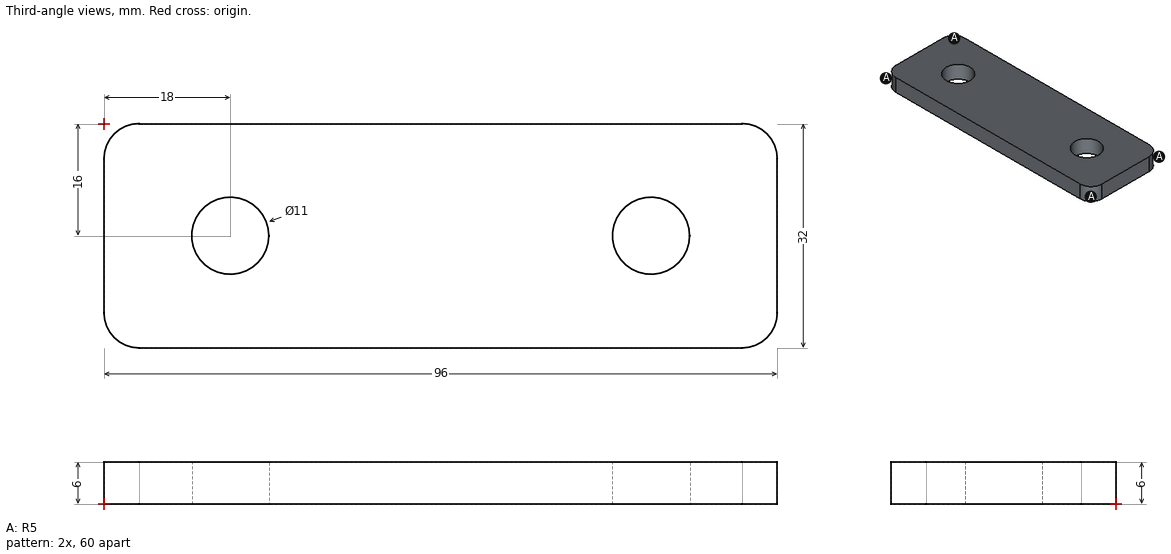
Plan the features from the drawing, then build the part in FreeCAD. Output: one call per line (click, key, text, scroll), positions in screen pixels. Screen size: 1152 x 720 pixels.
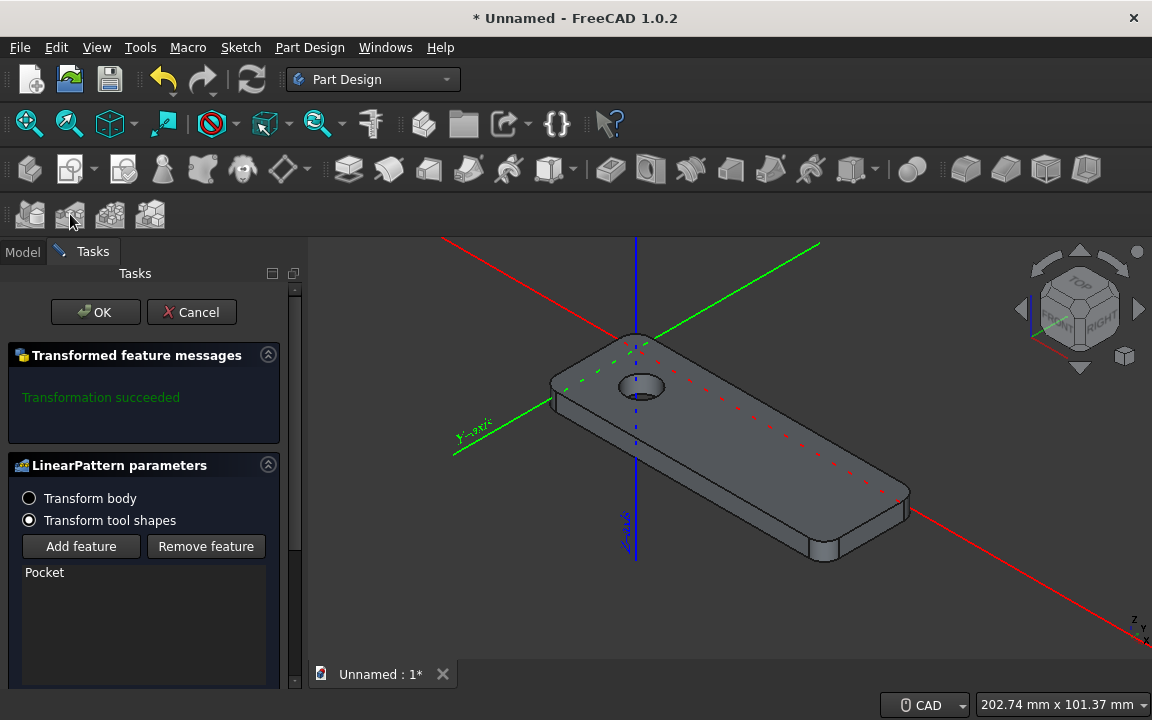
scroll(295, 486, down, 2)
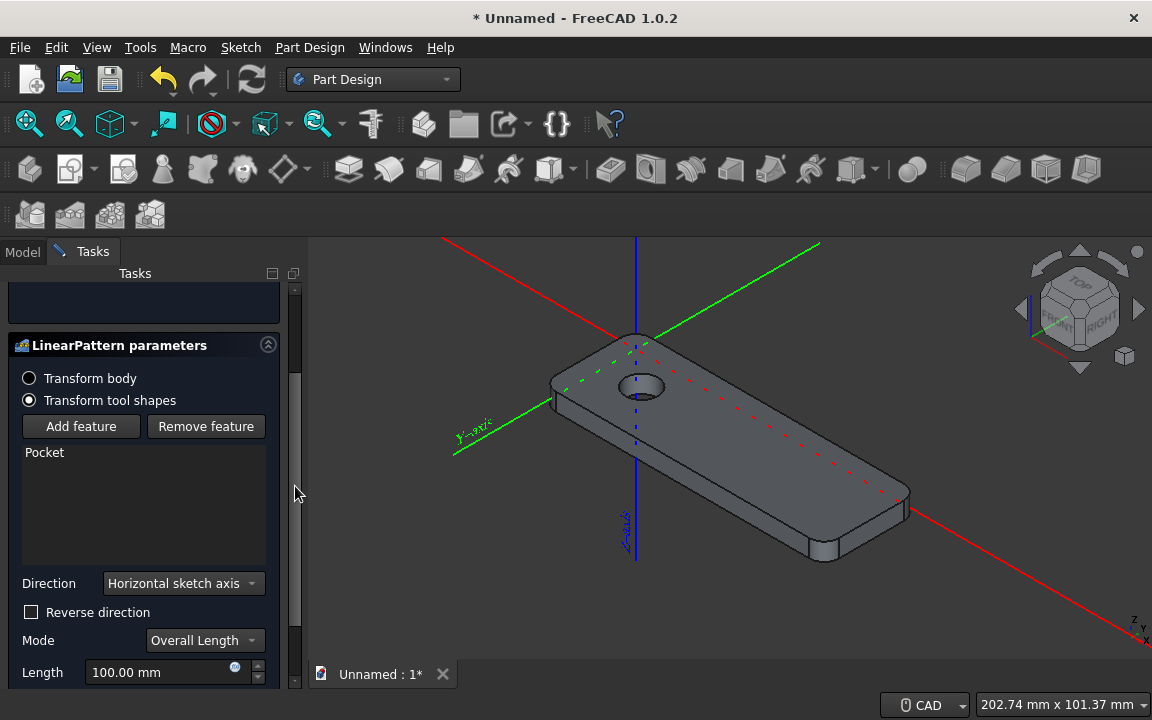
click(184, 584)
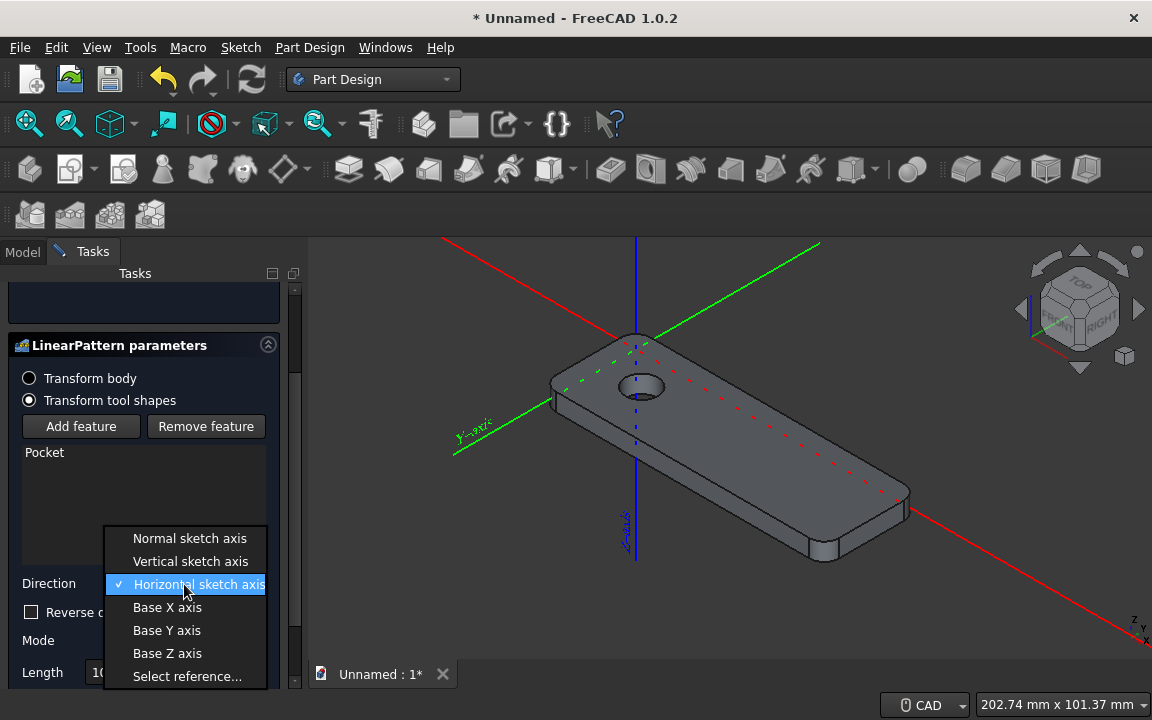
click(184, 608)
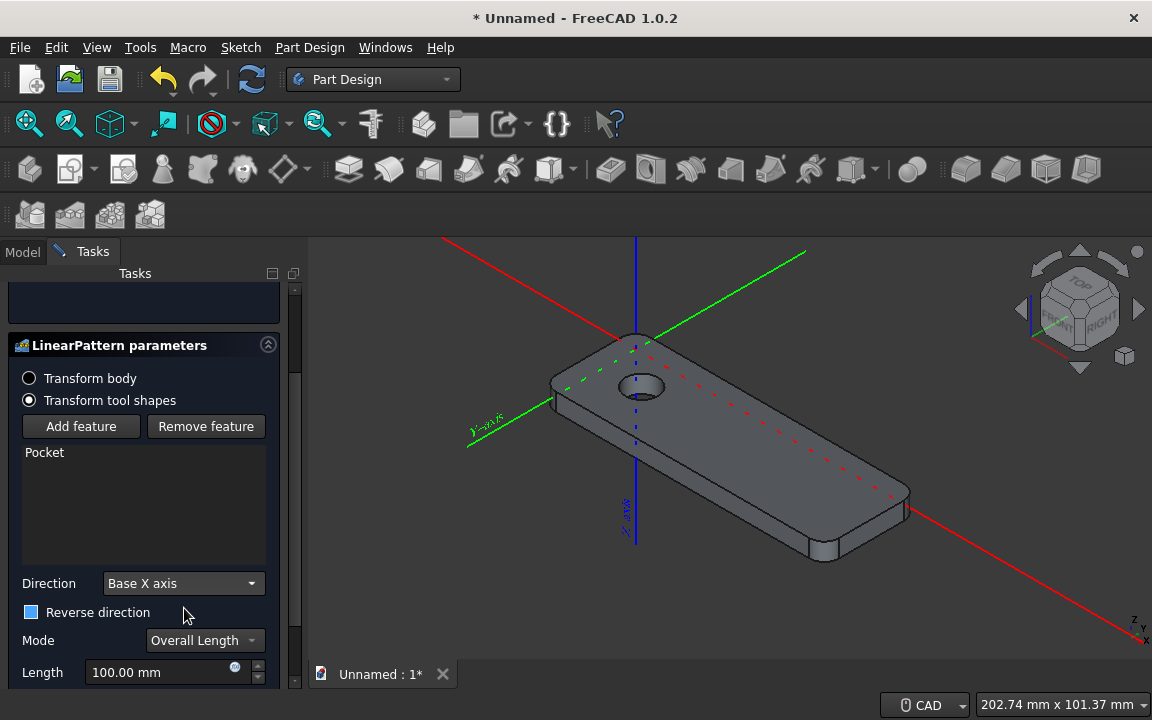
click(206, 640)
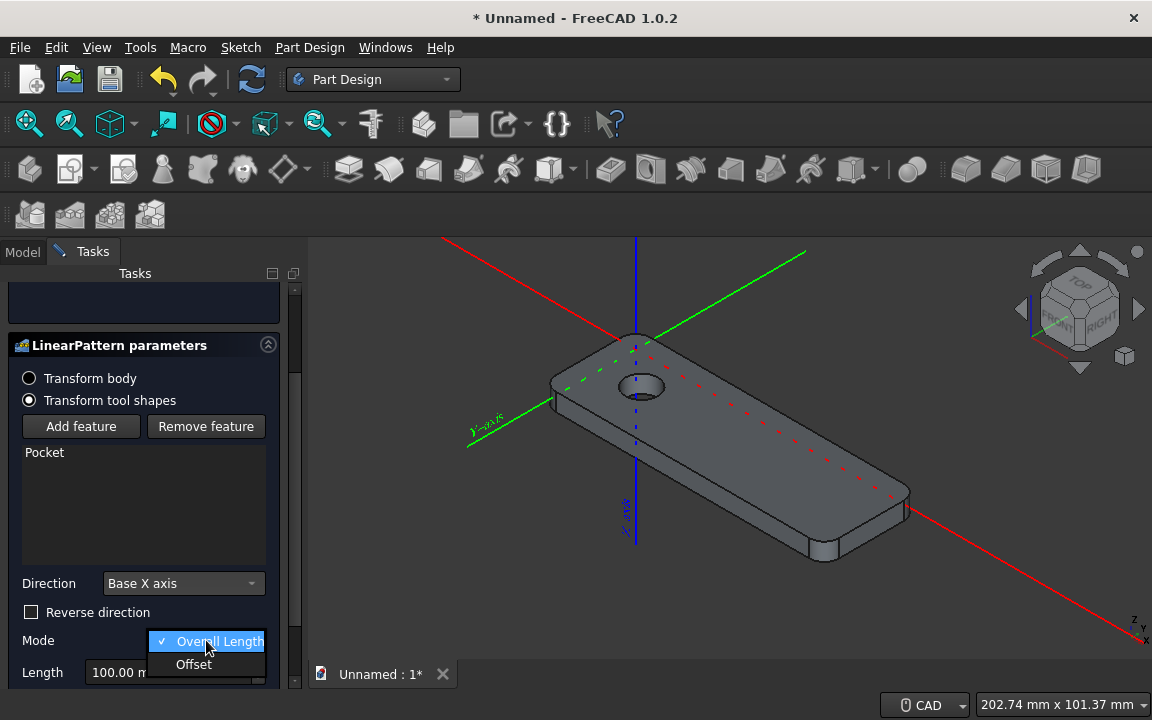
click(206, 664)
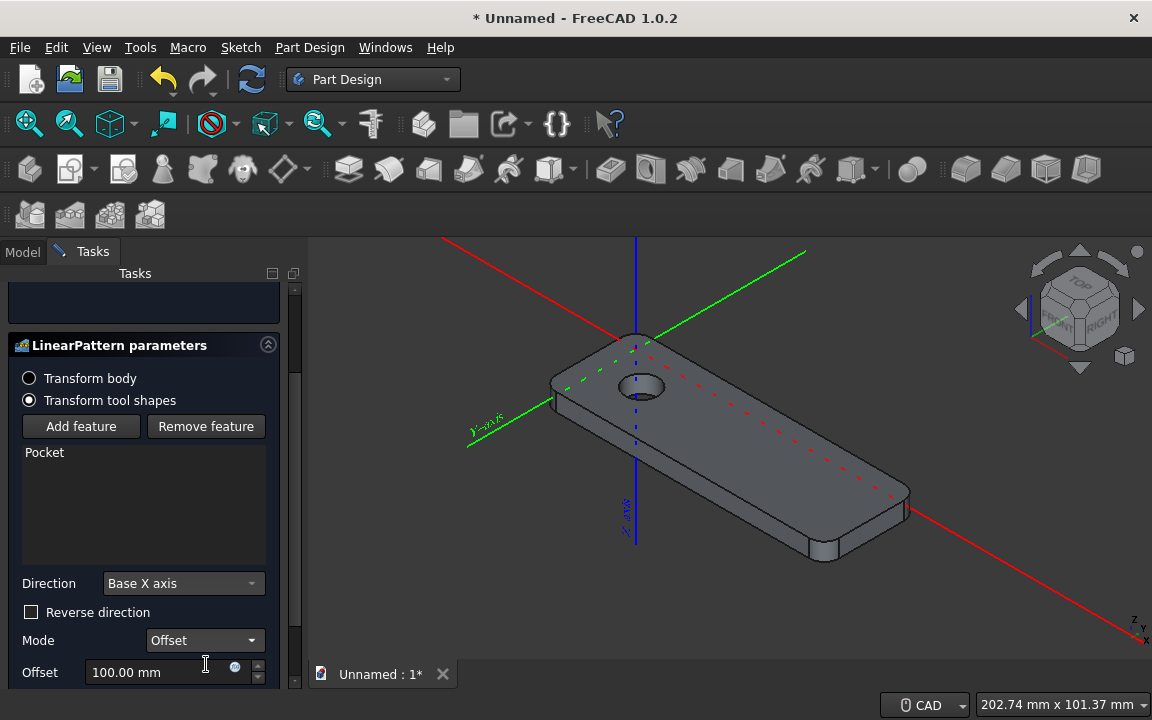
triple_click(168, 672)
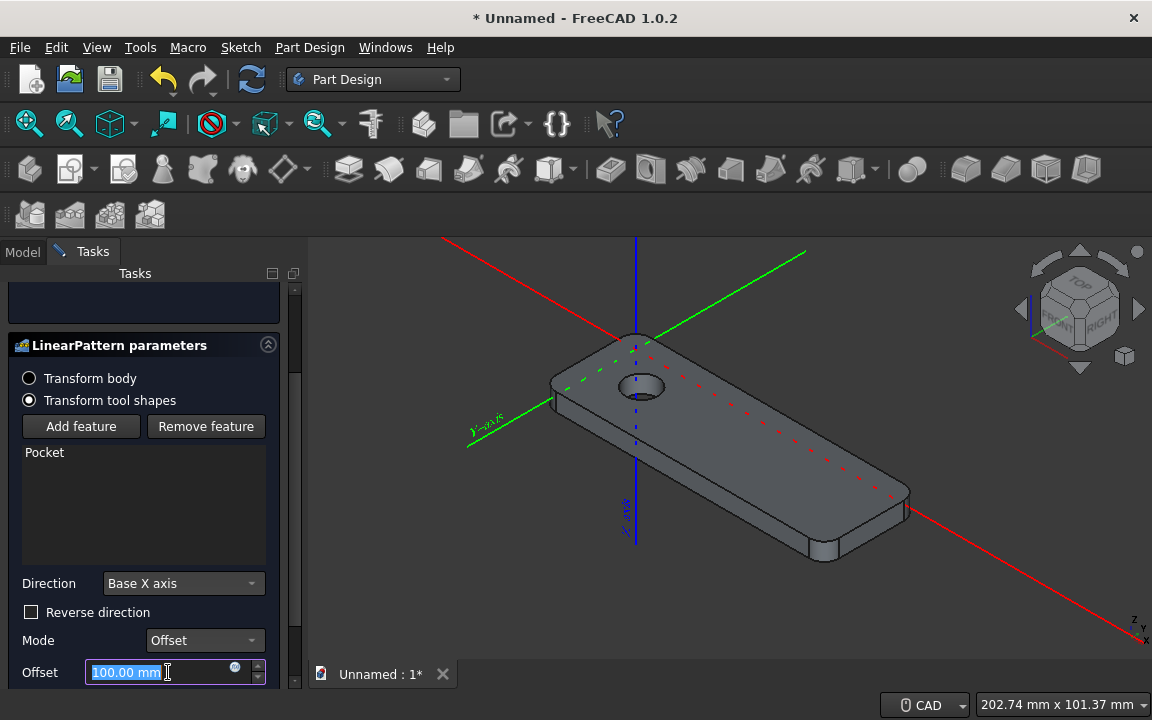
text(60)
key(Tab)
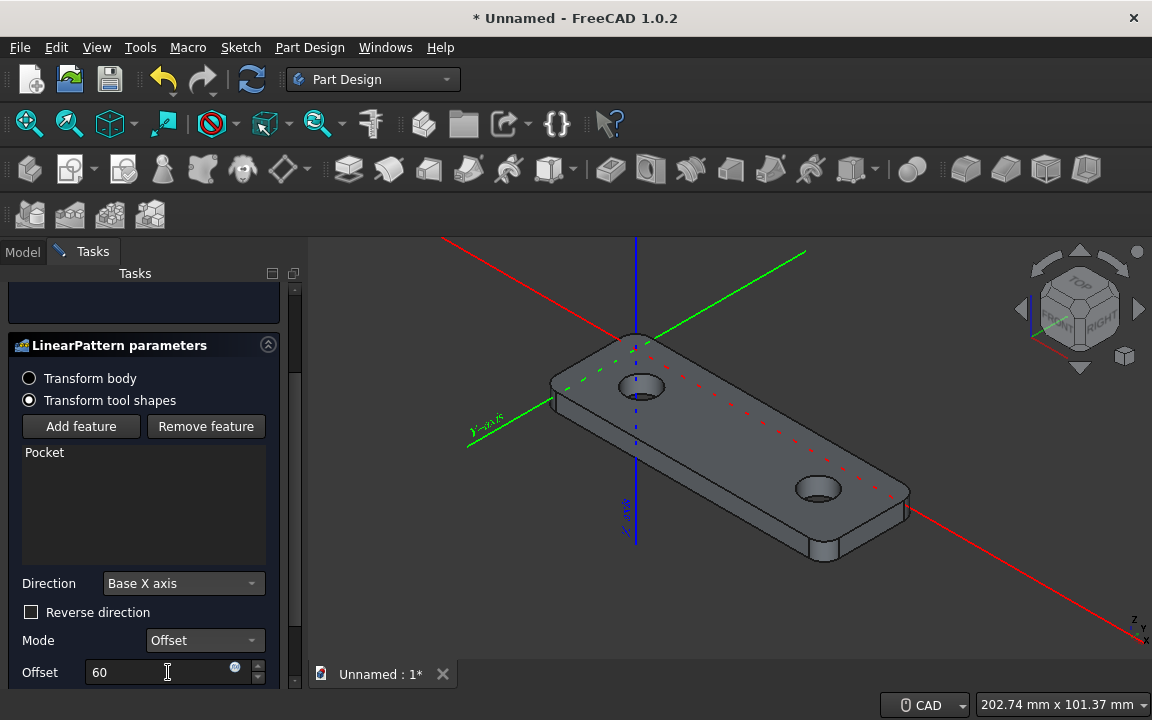
scroll(295, 486, down, 2)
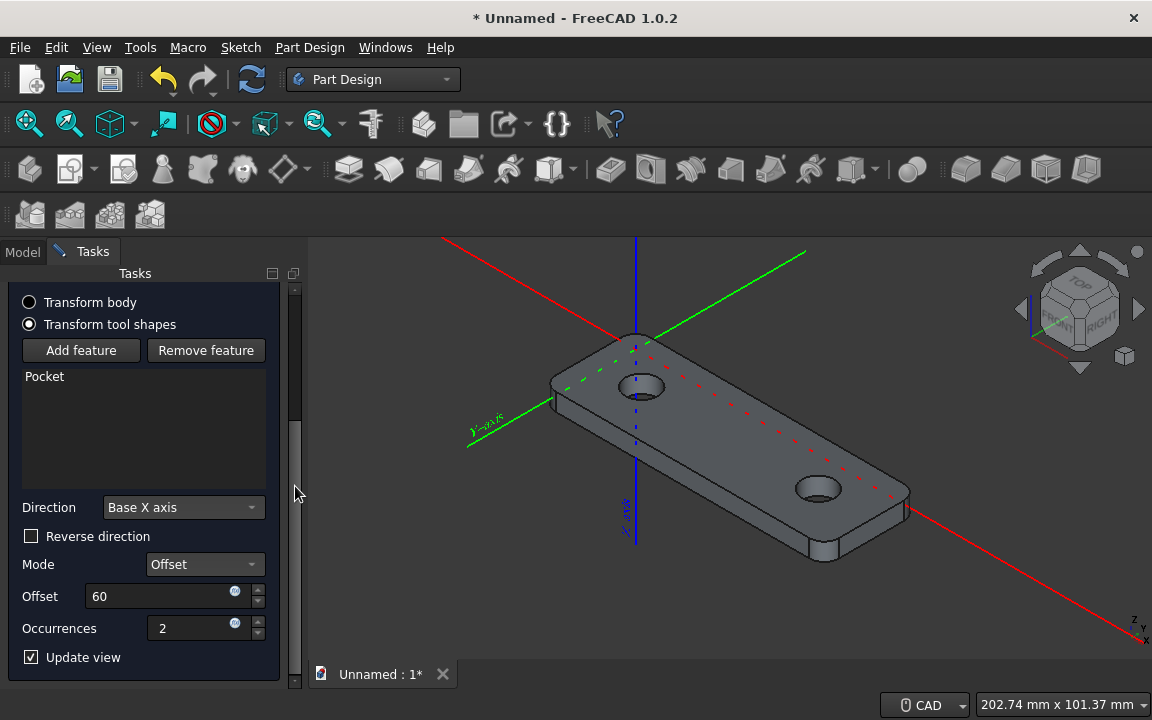
triple_click(198, 628)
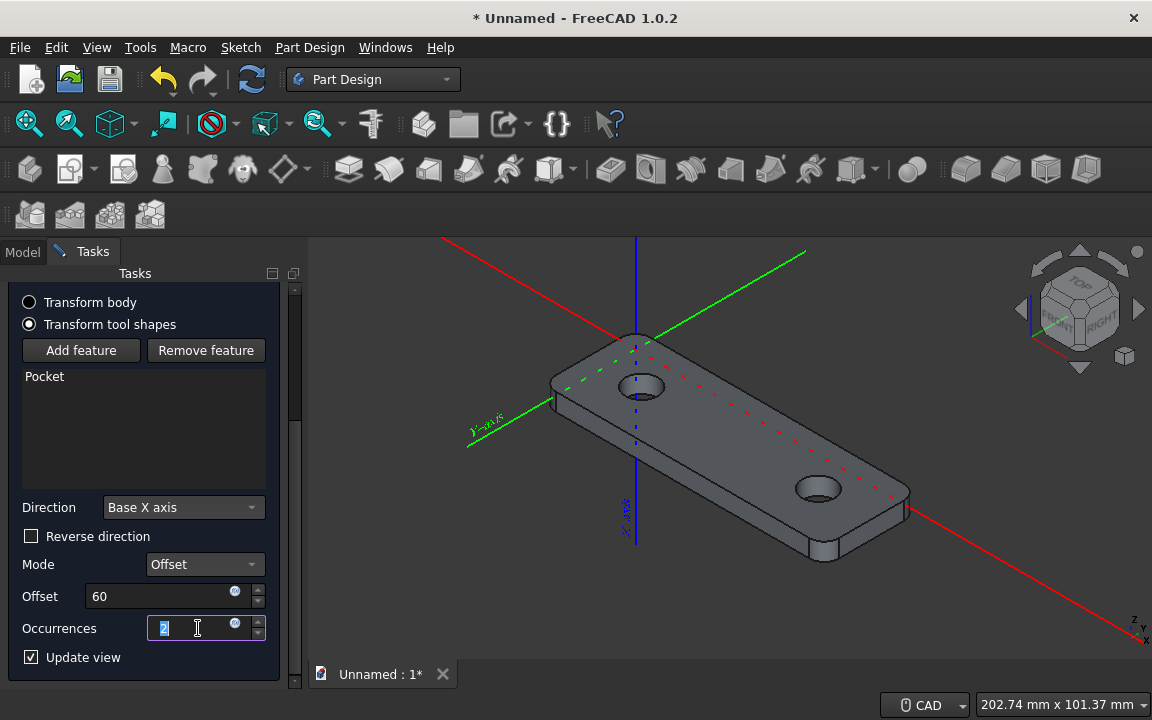
text(2)
key(Tab)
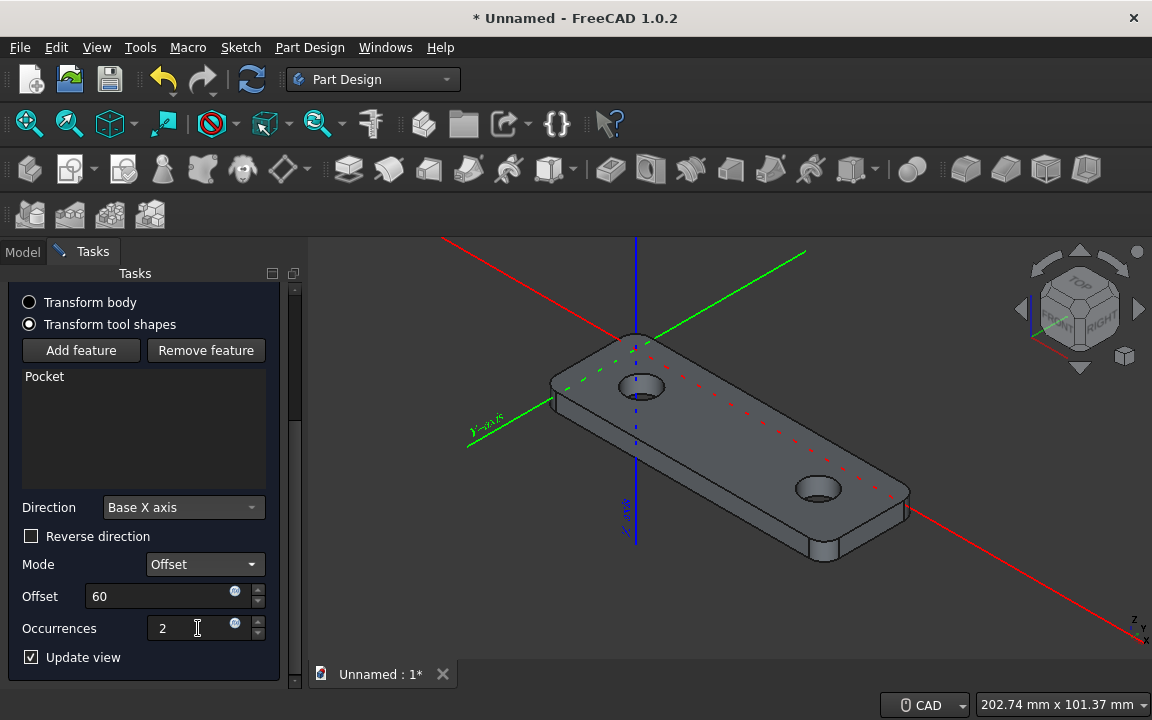
scroll(295, 486, up, 5)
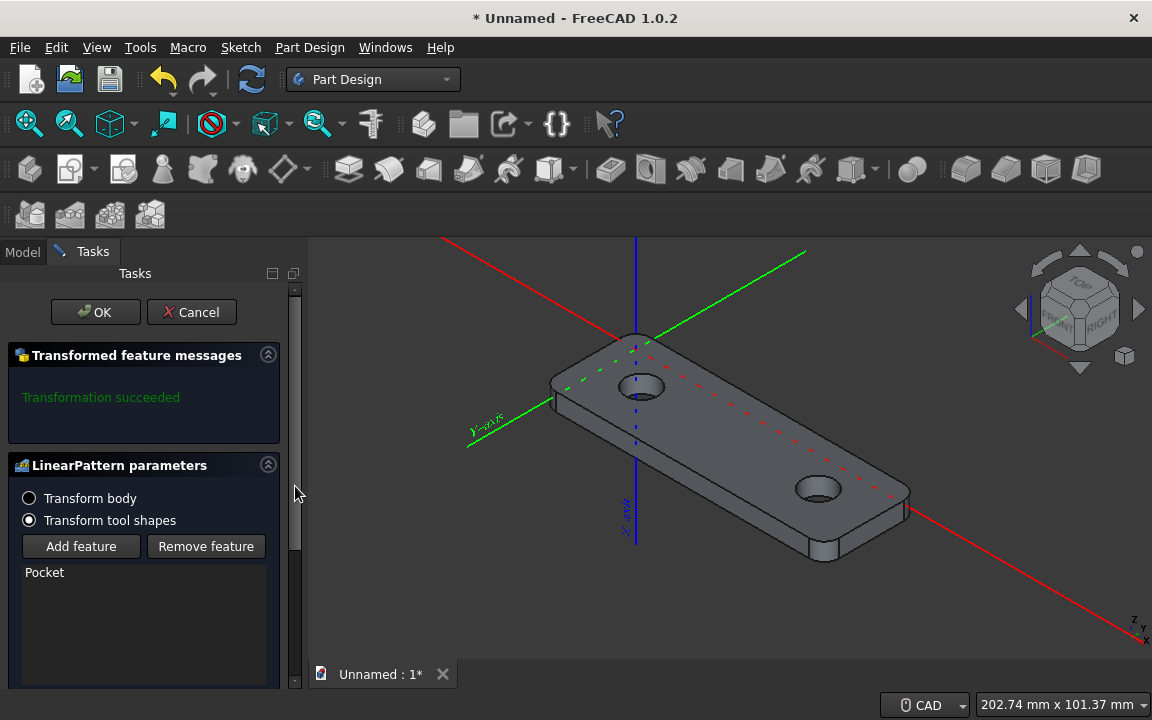
click(96, 312)